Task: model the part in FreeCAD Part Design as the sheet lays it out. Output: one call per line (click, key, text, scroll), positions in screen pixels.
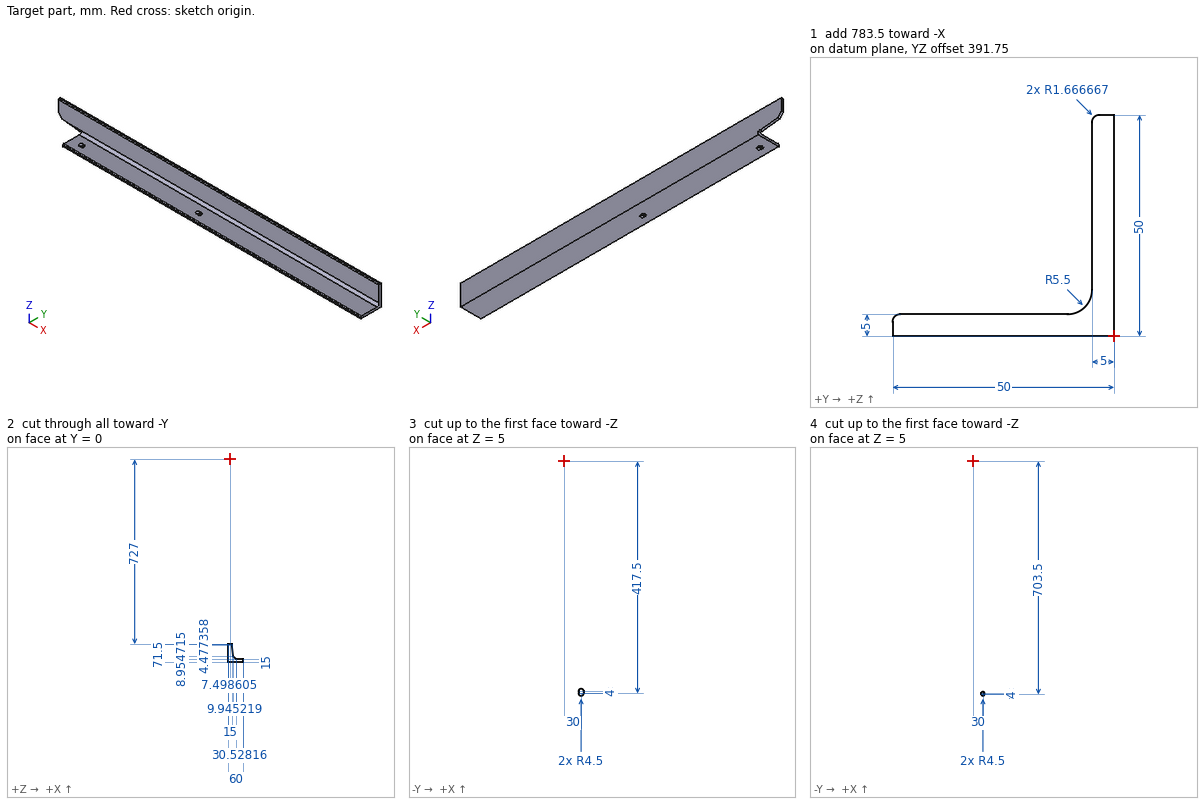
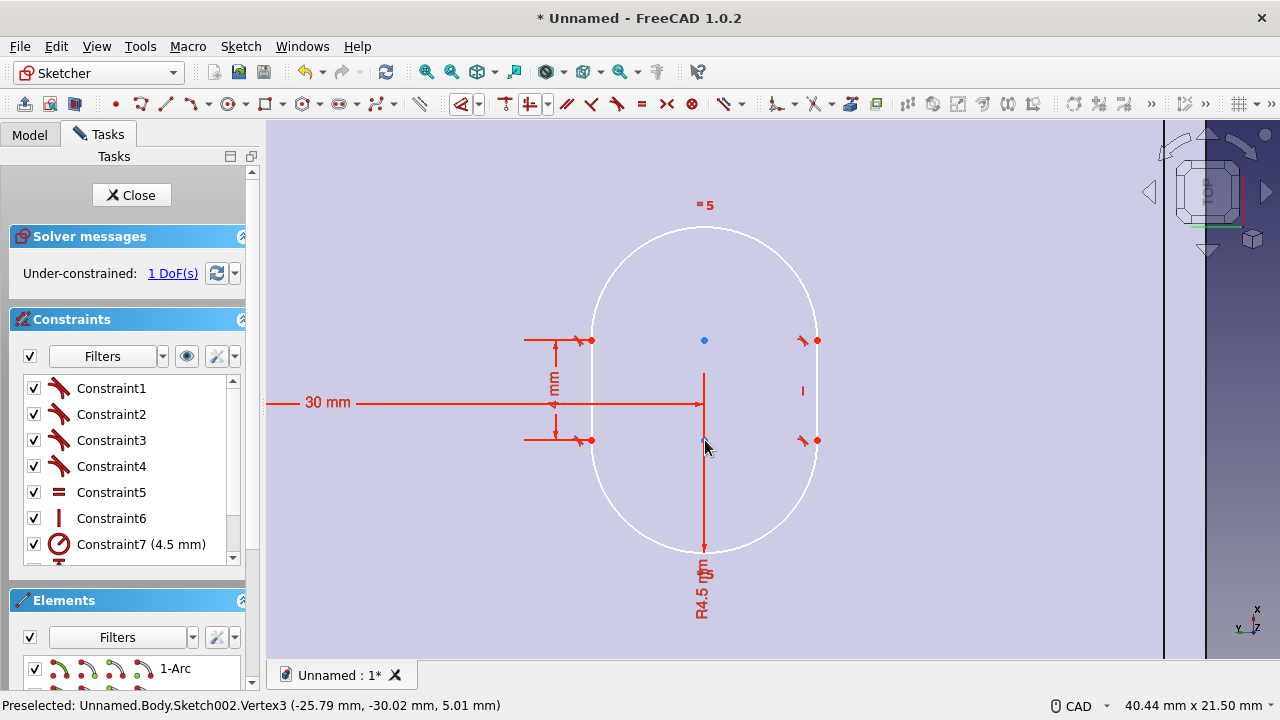
click(592, 440)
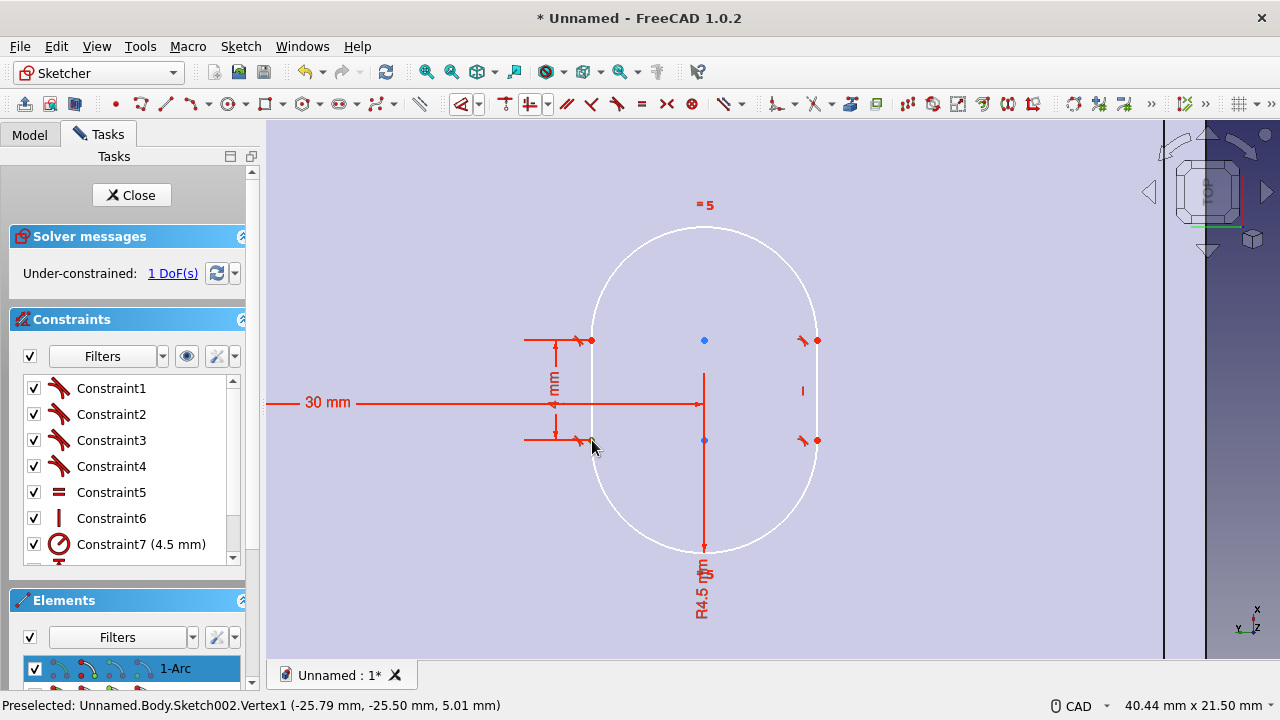
click(478, 104)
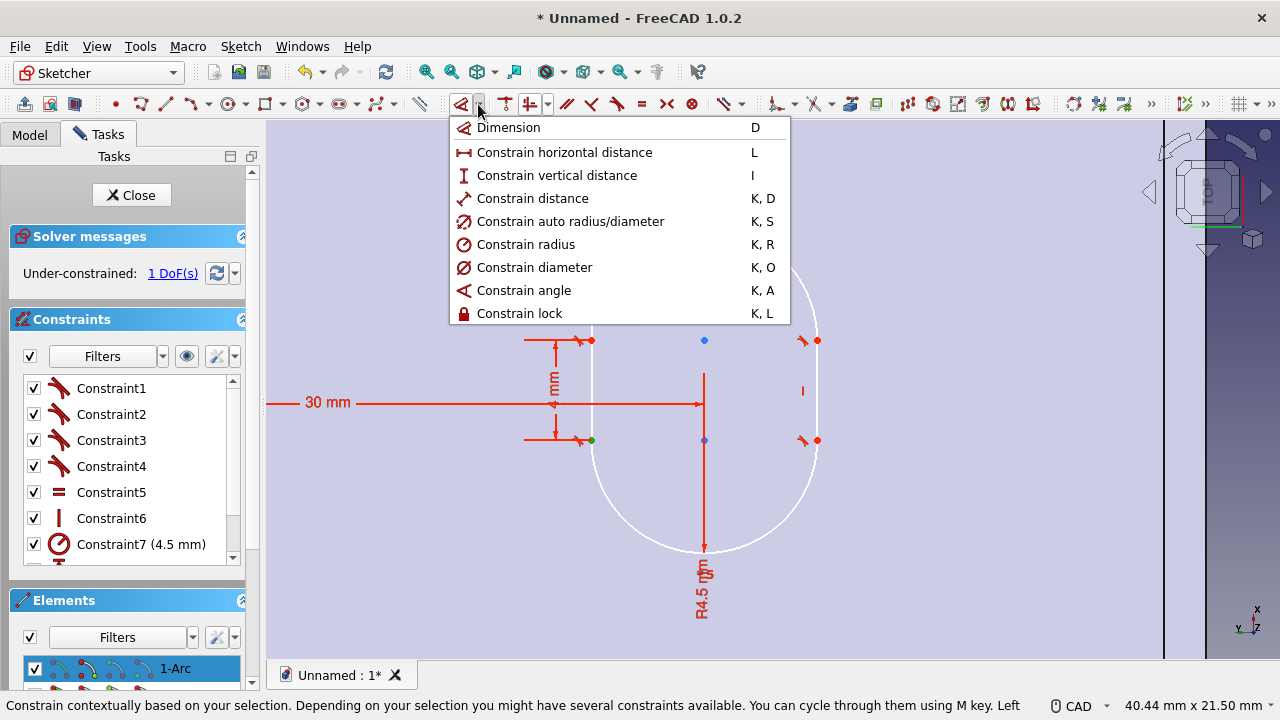
click(620, 176)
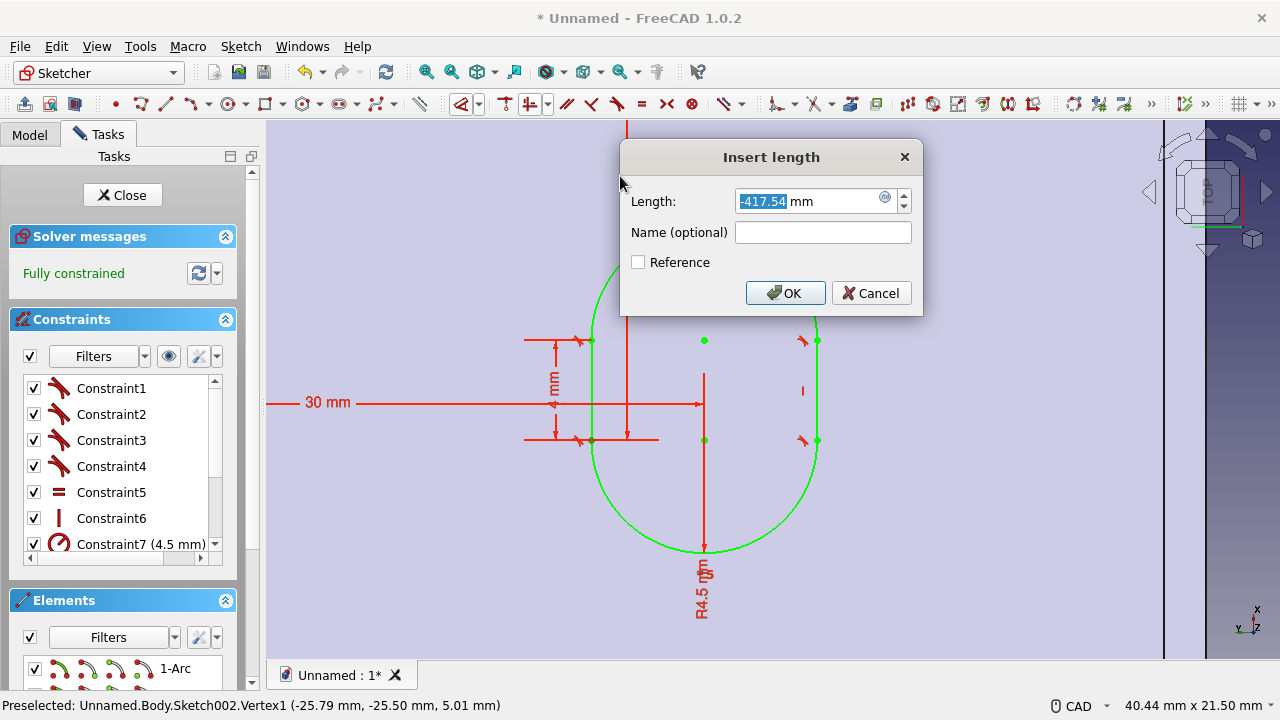
text(-417.5)
key(Return)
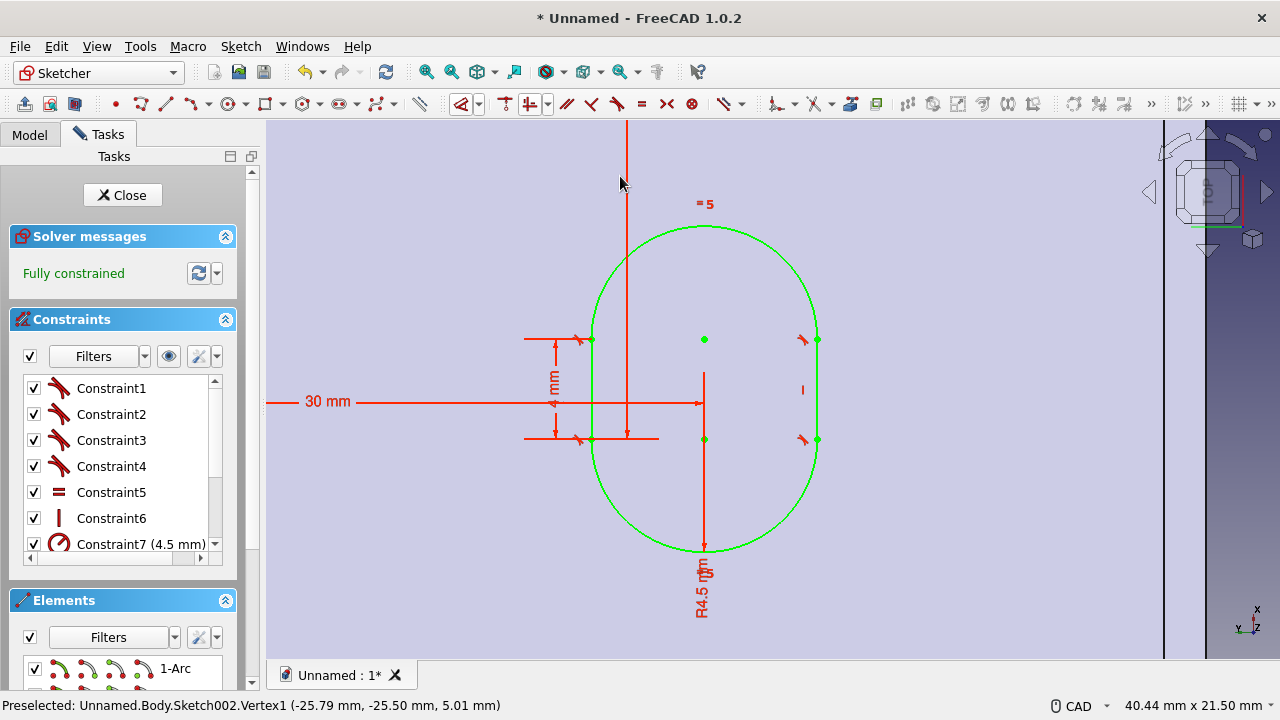
click(123, 195)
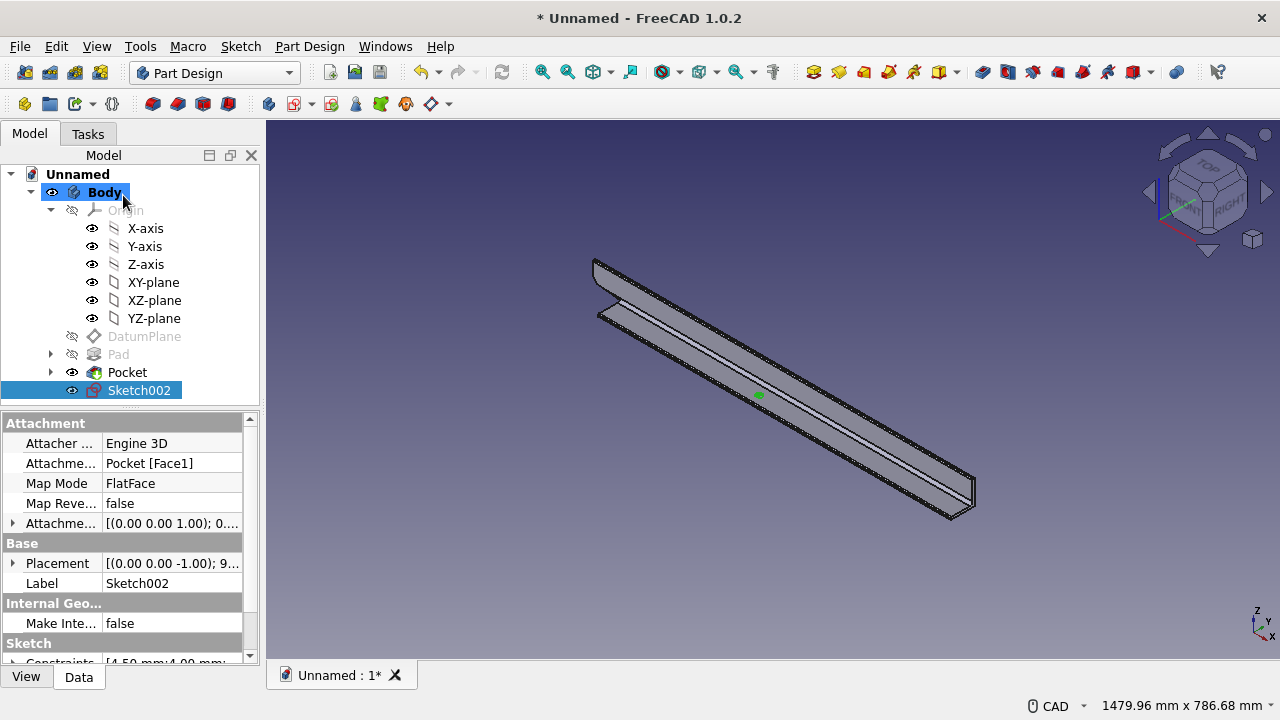
click(983, 72)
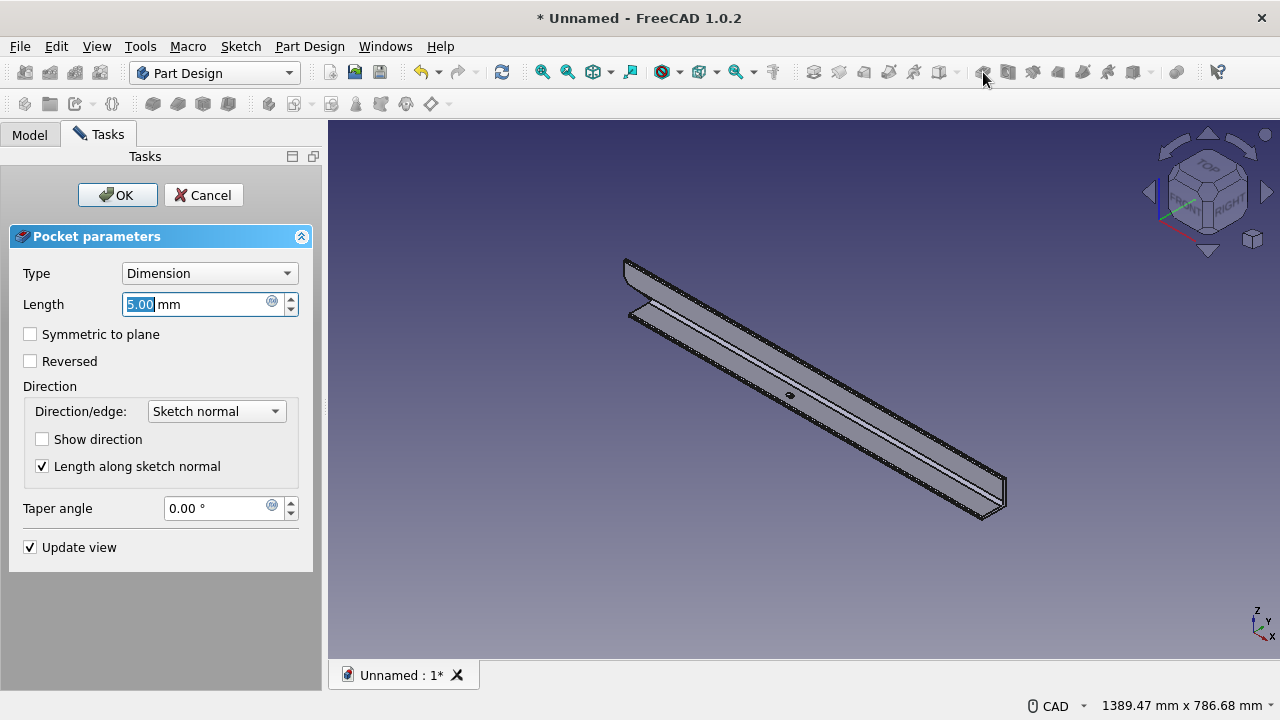
click(210, 274)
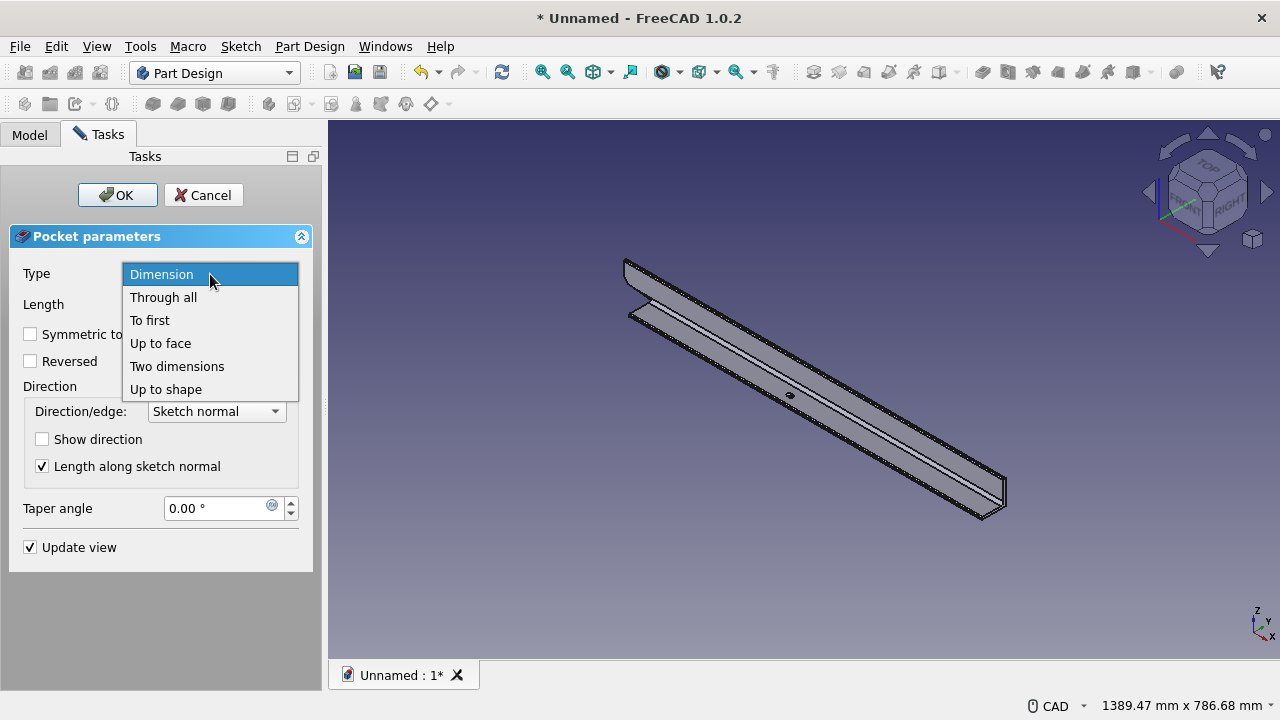
click(208, 320)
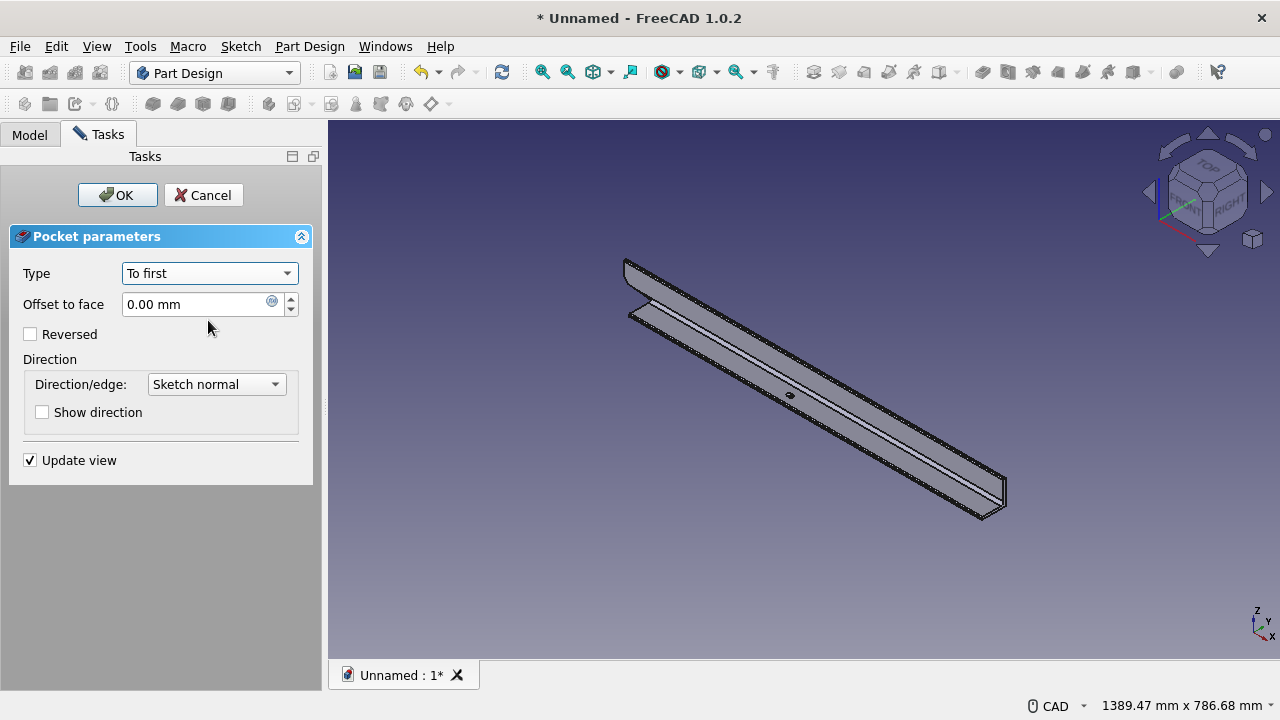
click(118, 195)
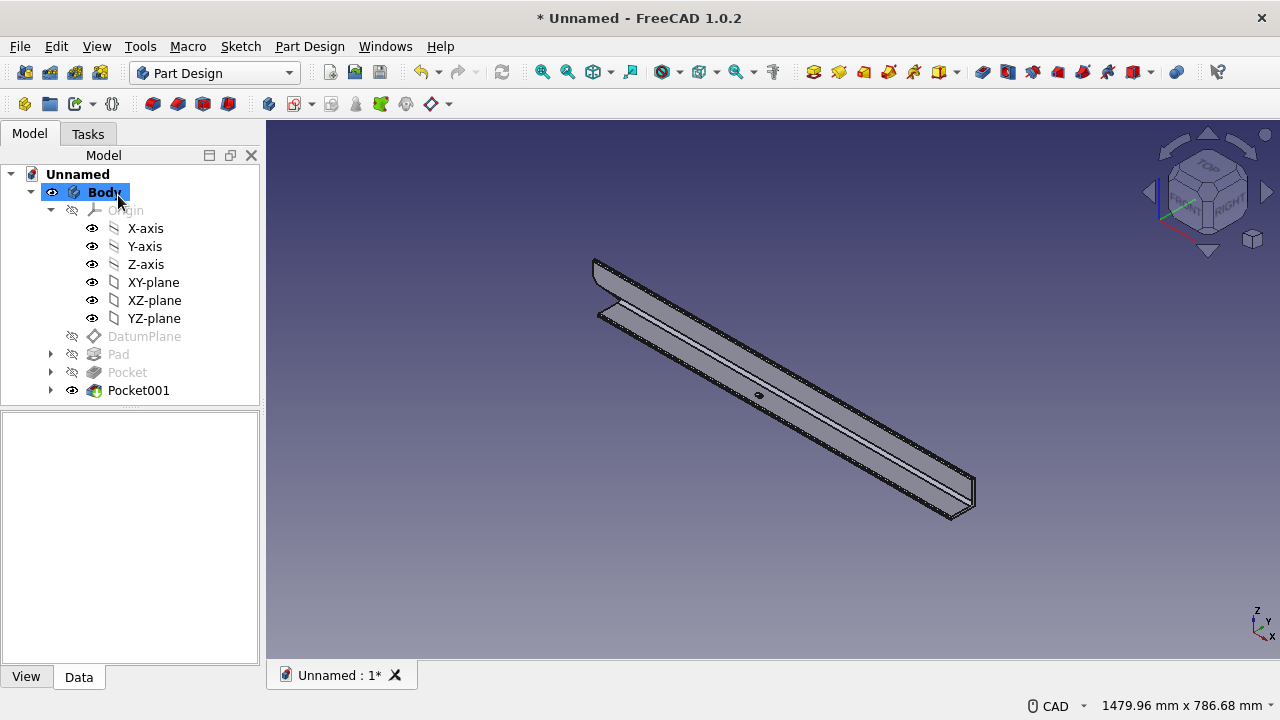
click(785, 409)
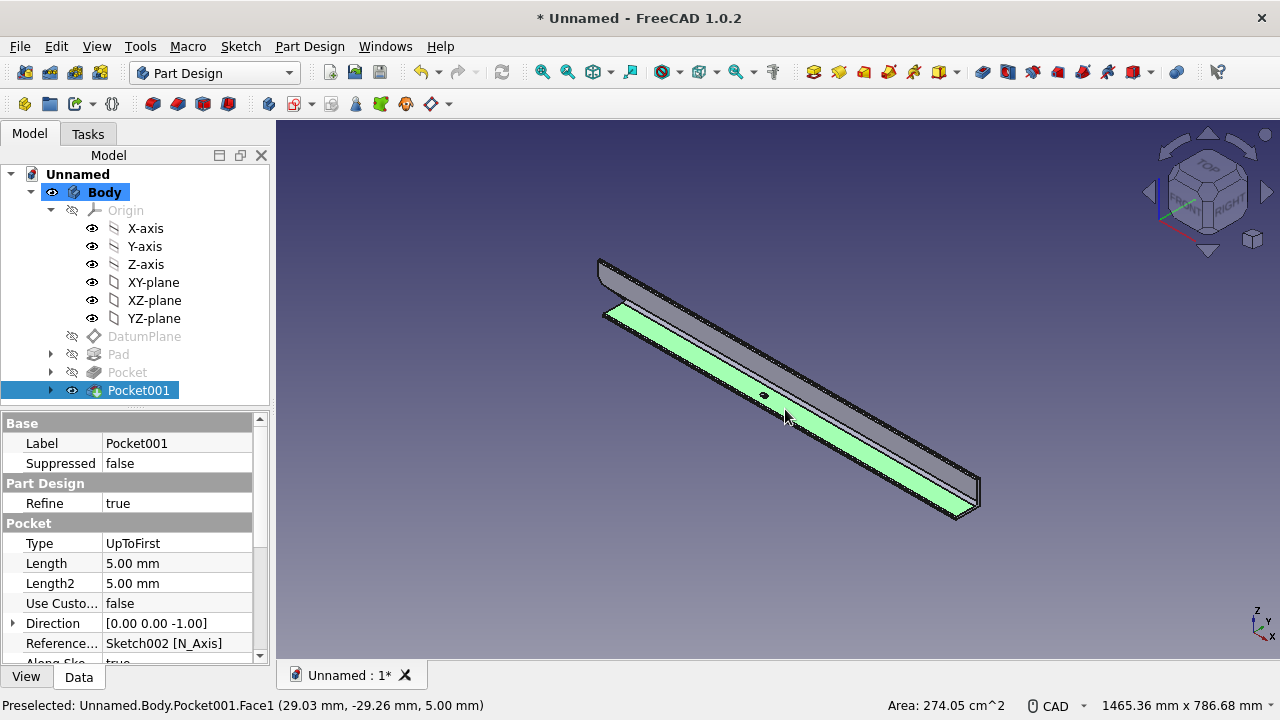
click(294, 104)